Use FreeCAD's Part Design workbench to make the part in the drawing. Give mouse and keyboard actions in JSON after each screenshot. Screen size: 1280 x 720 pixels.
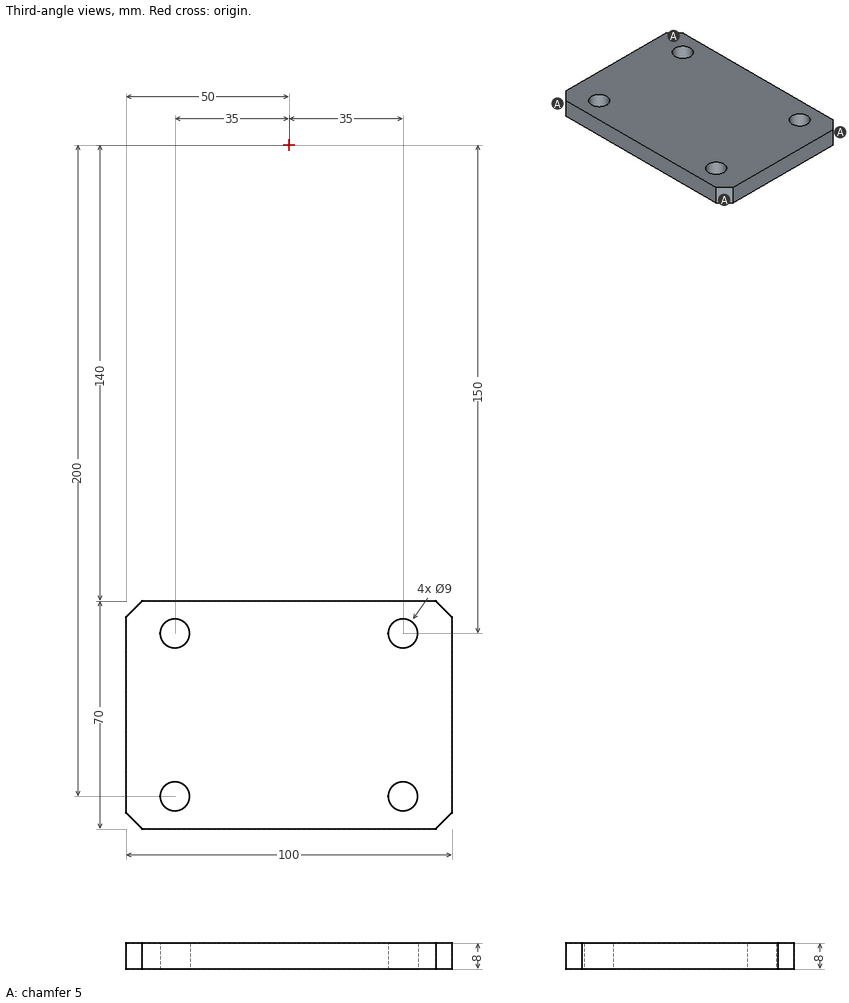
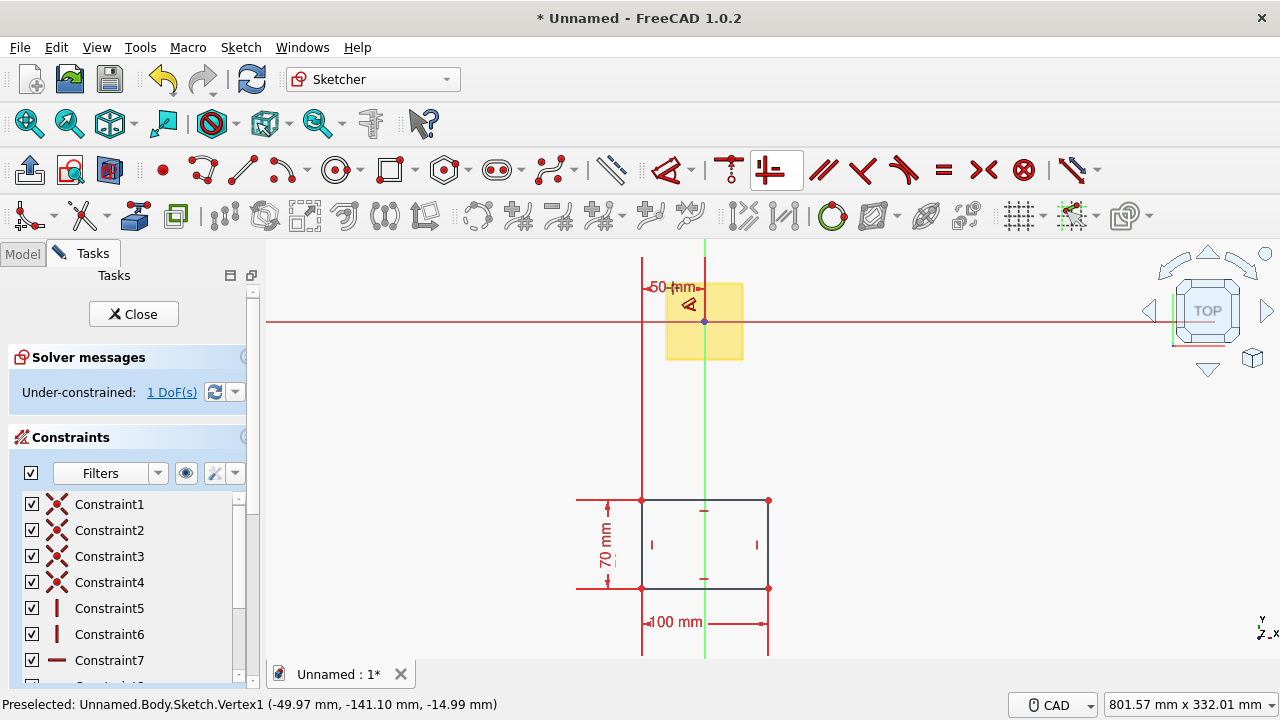
{"action": "left_click", "coordinate": [642, 500]}
{"action": "left_click", "coordinate": [608, 411]}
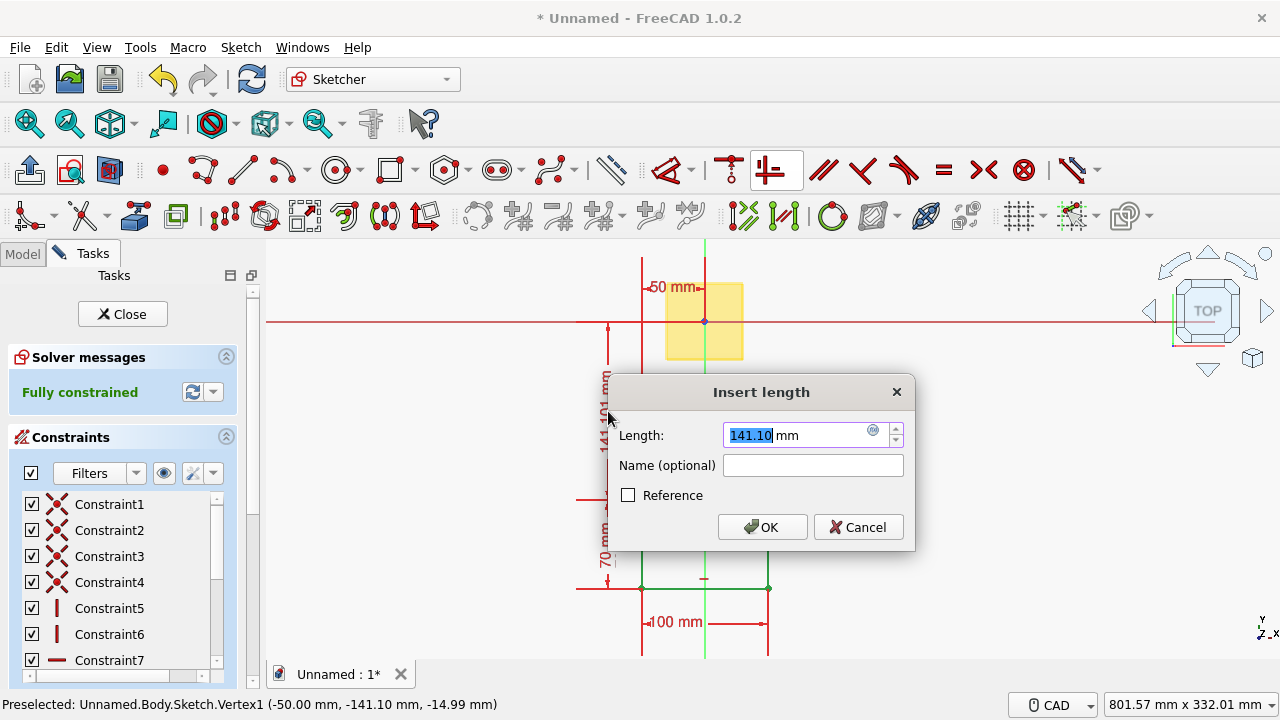
{"action": "type", "text": "140"}
{"action": "key", "text": "Return"}
{"action": "key", "text": "Escape"}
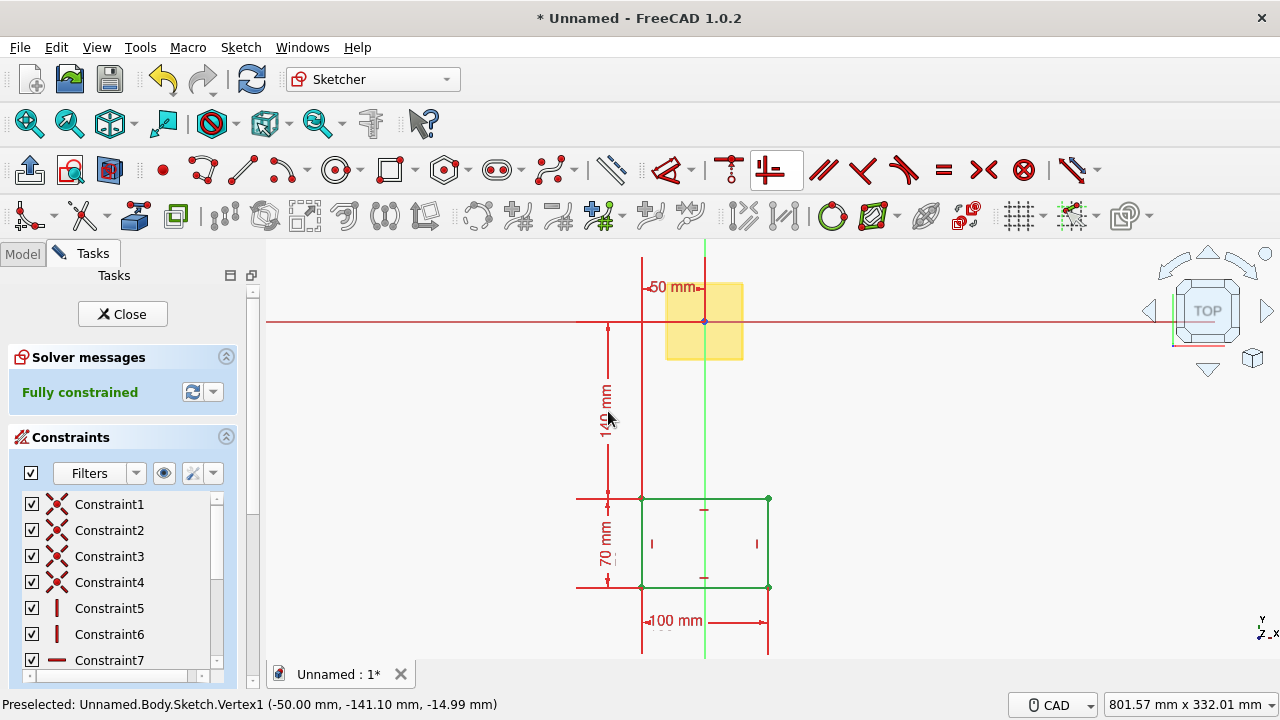
{"action": "left_click", "coordinate": [123, 314]}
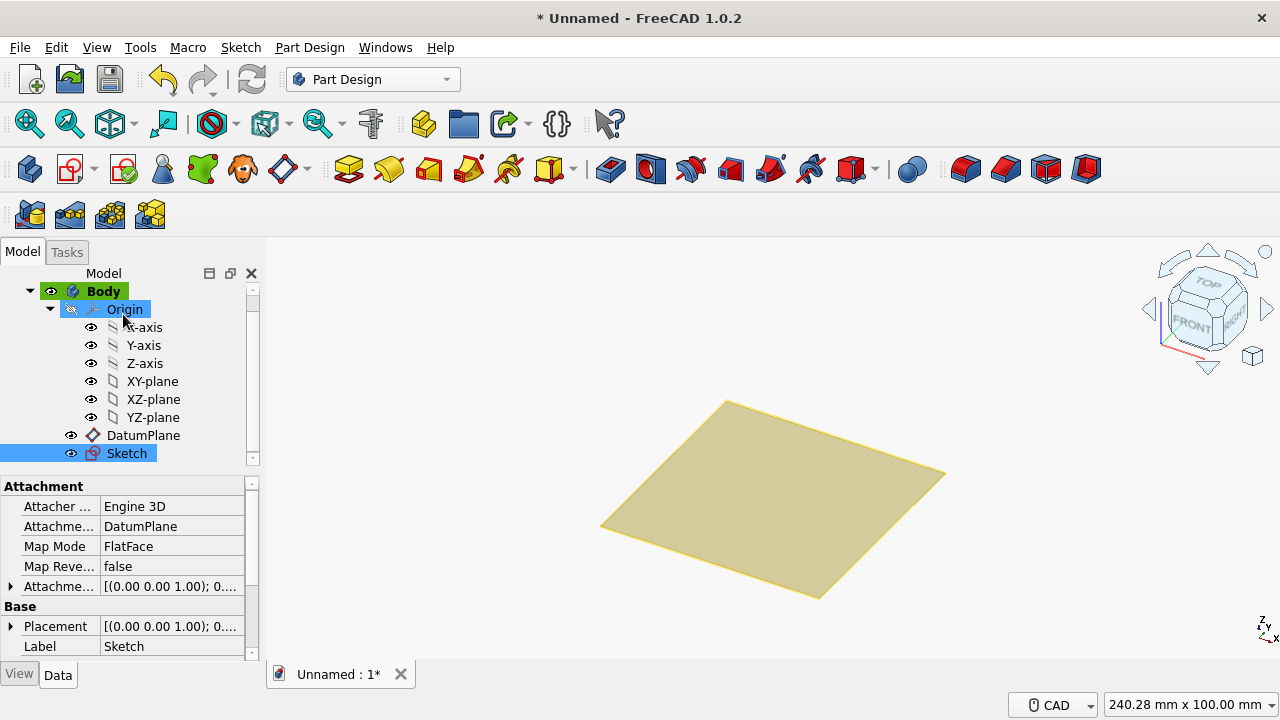
{"action": "left_click", "coordinate": [350, 170]}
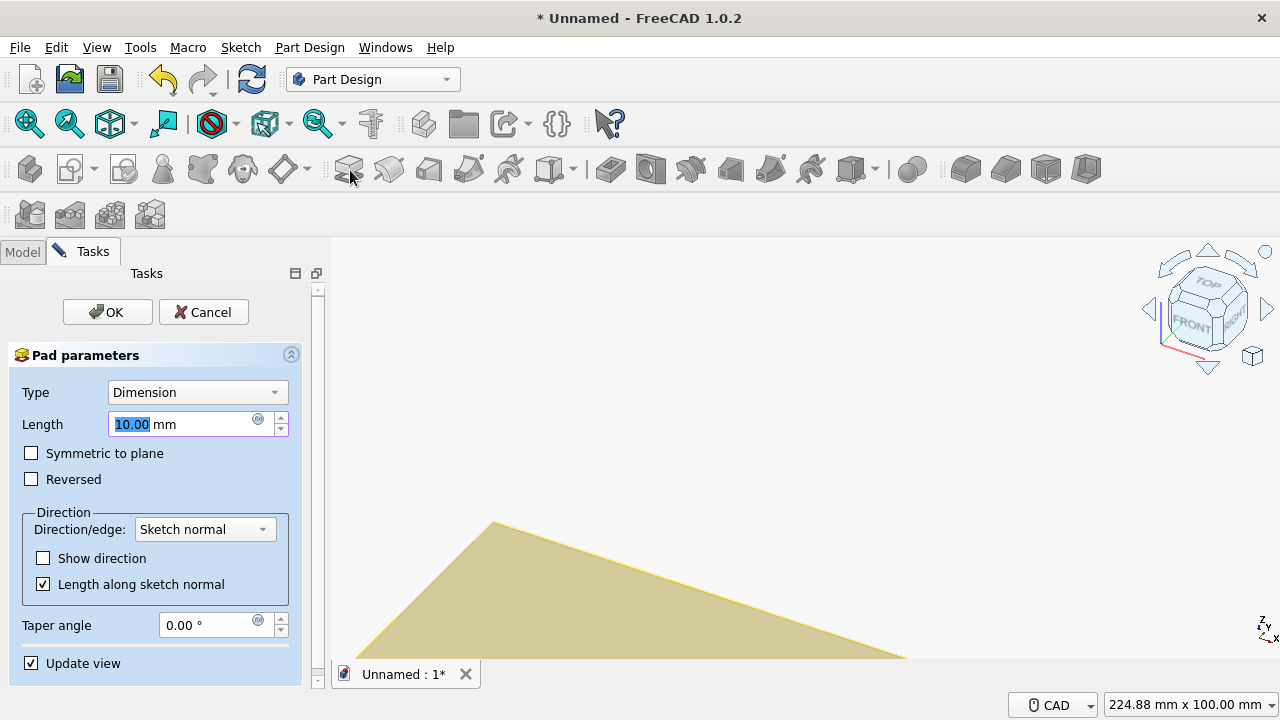
{"action": "type", "text": "8"}
{"action": "key", "text": "Tab"}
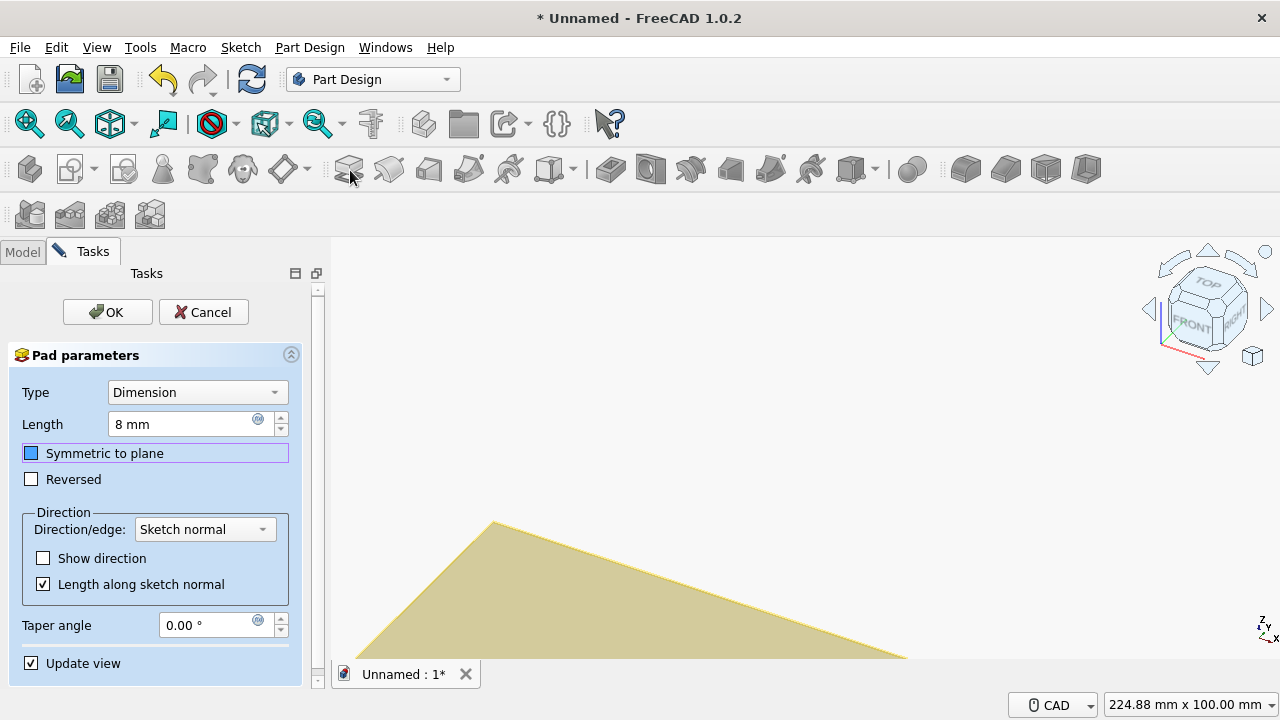
{"action": "left_click", "coordinate": [30, 479]}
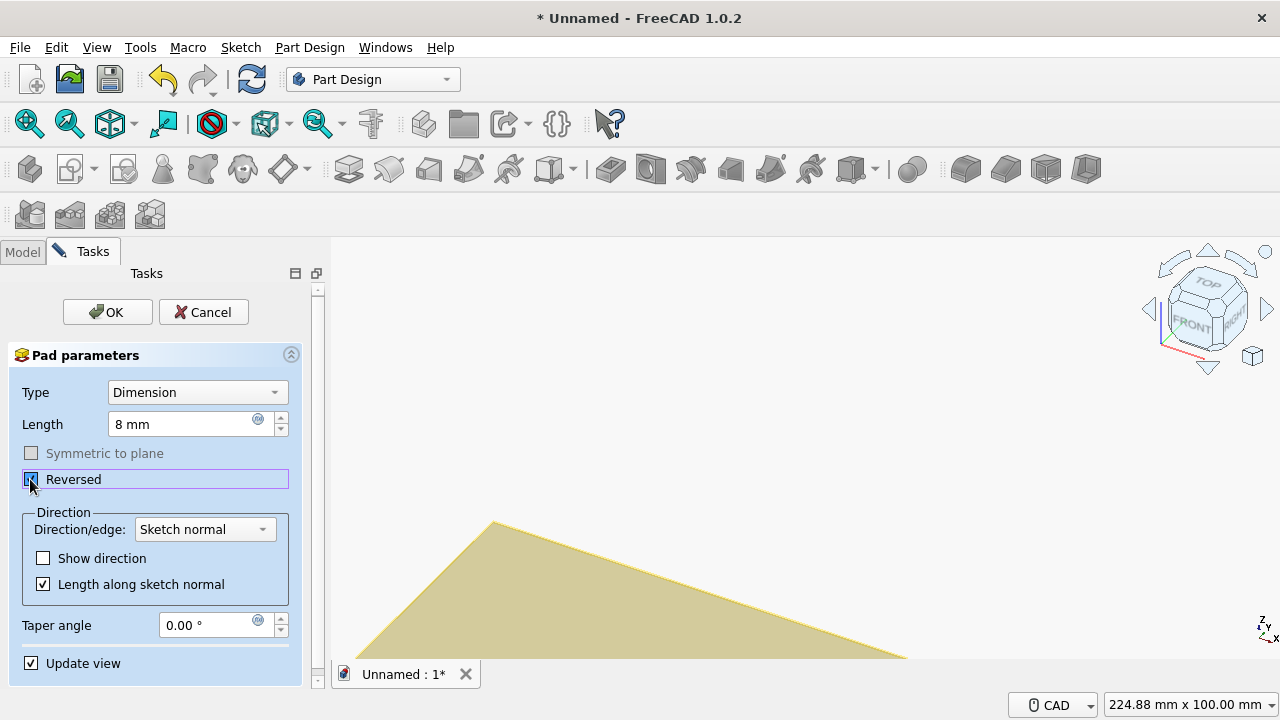
{"action": "left_click", "coordinate": [108, 312]}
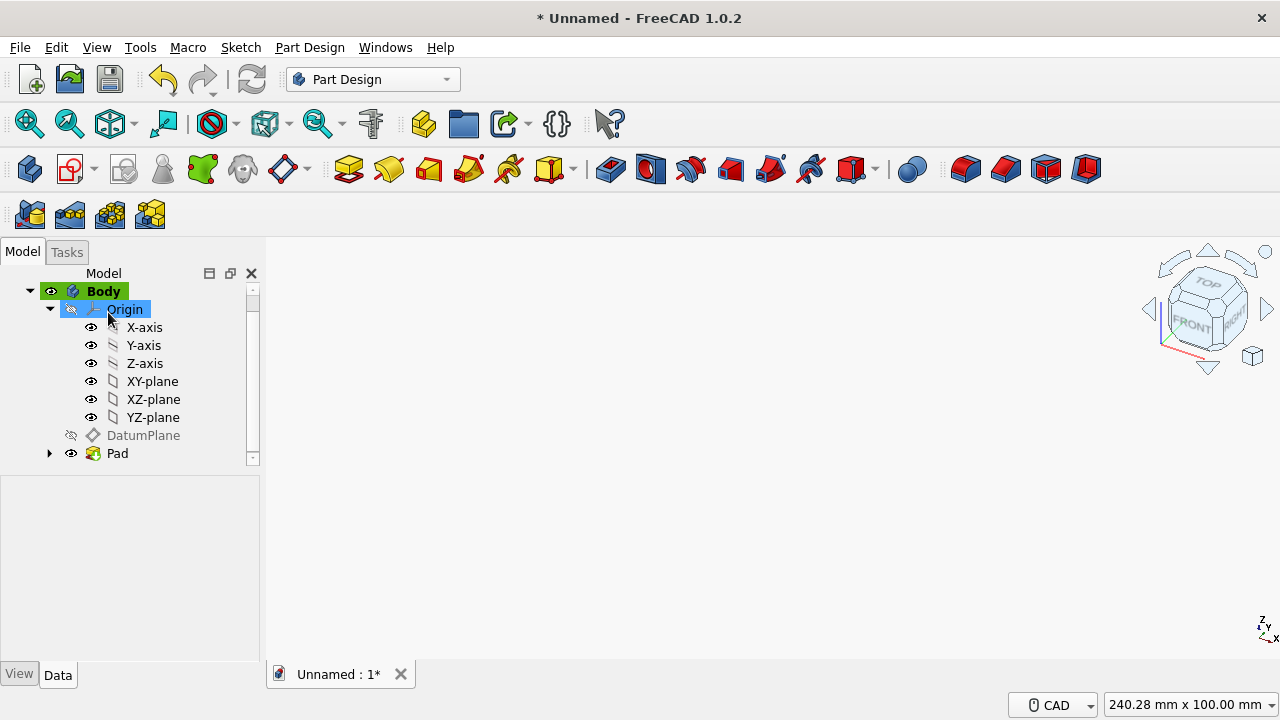
{"action": "left_click", "coordinate": [30, 124]}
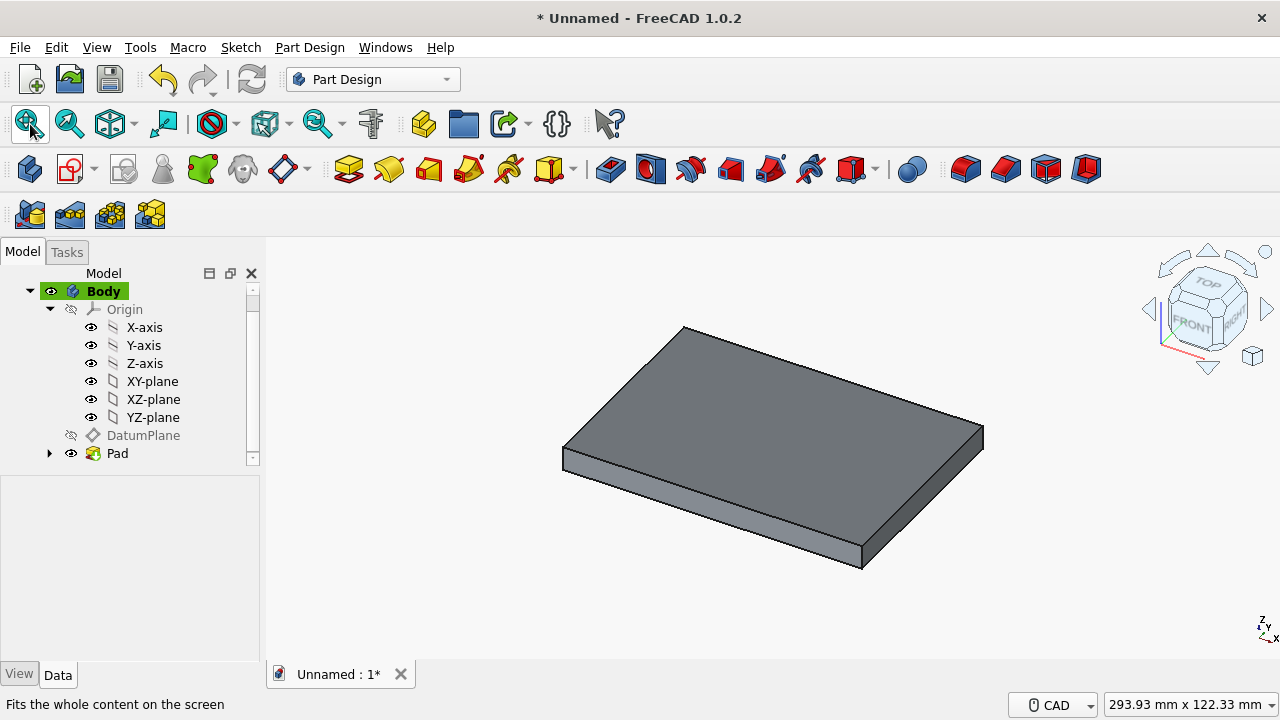
{"action": "key", "text": "5"}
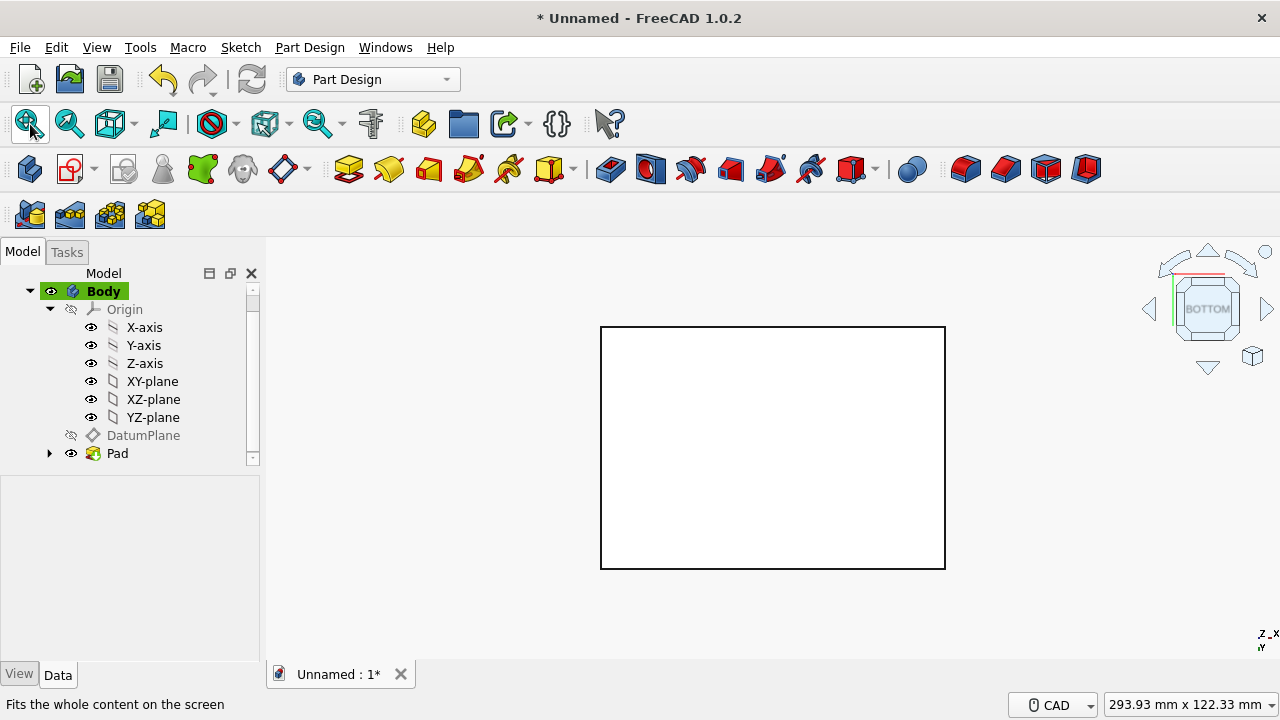
{"action": "left_click", "coordinate": [822, 447]}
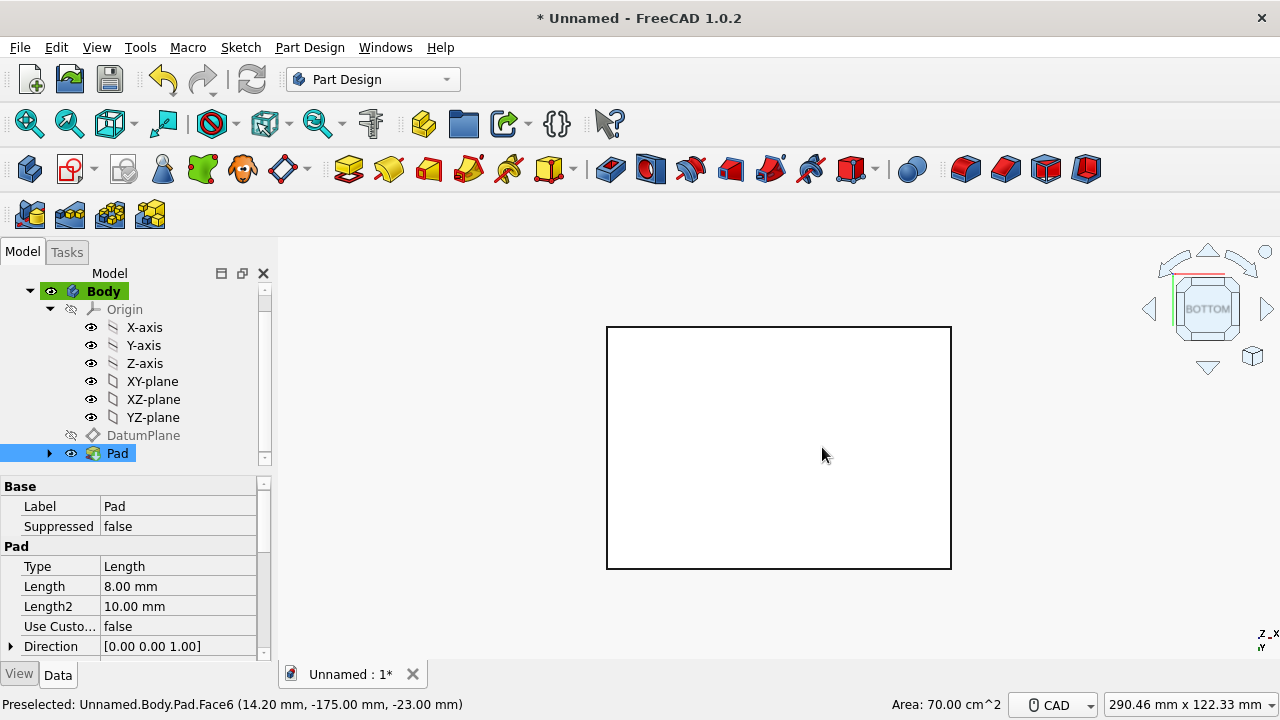
{"action": "left_click", "coordinate": [70, 170]}